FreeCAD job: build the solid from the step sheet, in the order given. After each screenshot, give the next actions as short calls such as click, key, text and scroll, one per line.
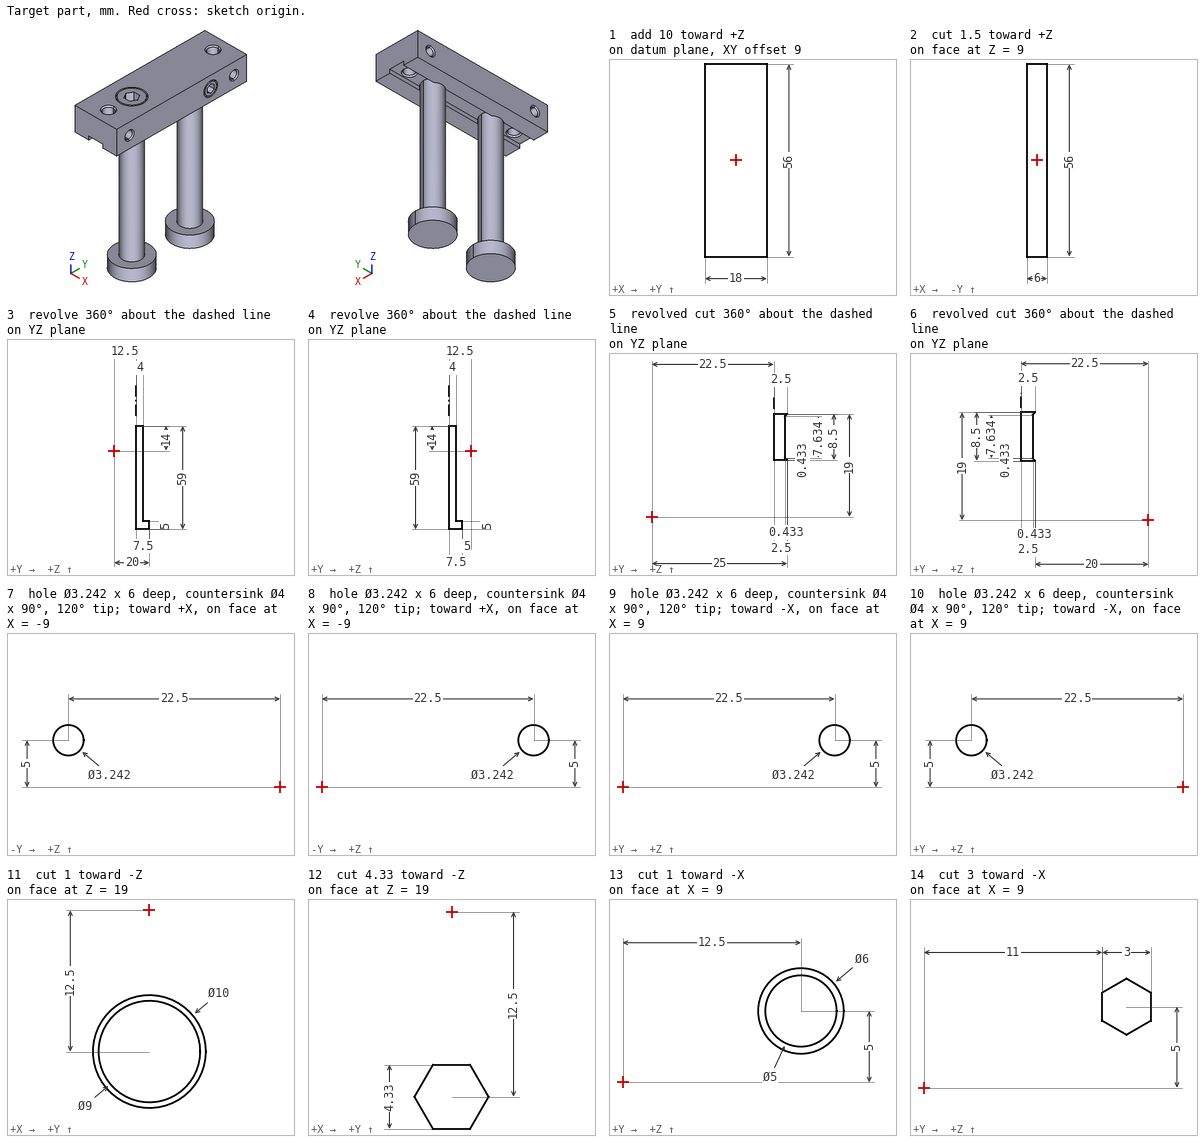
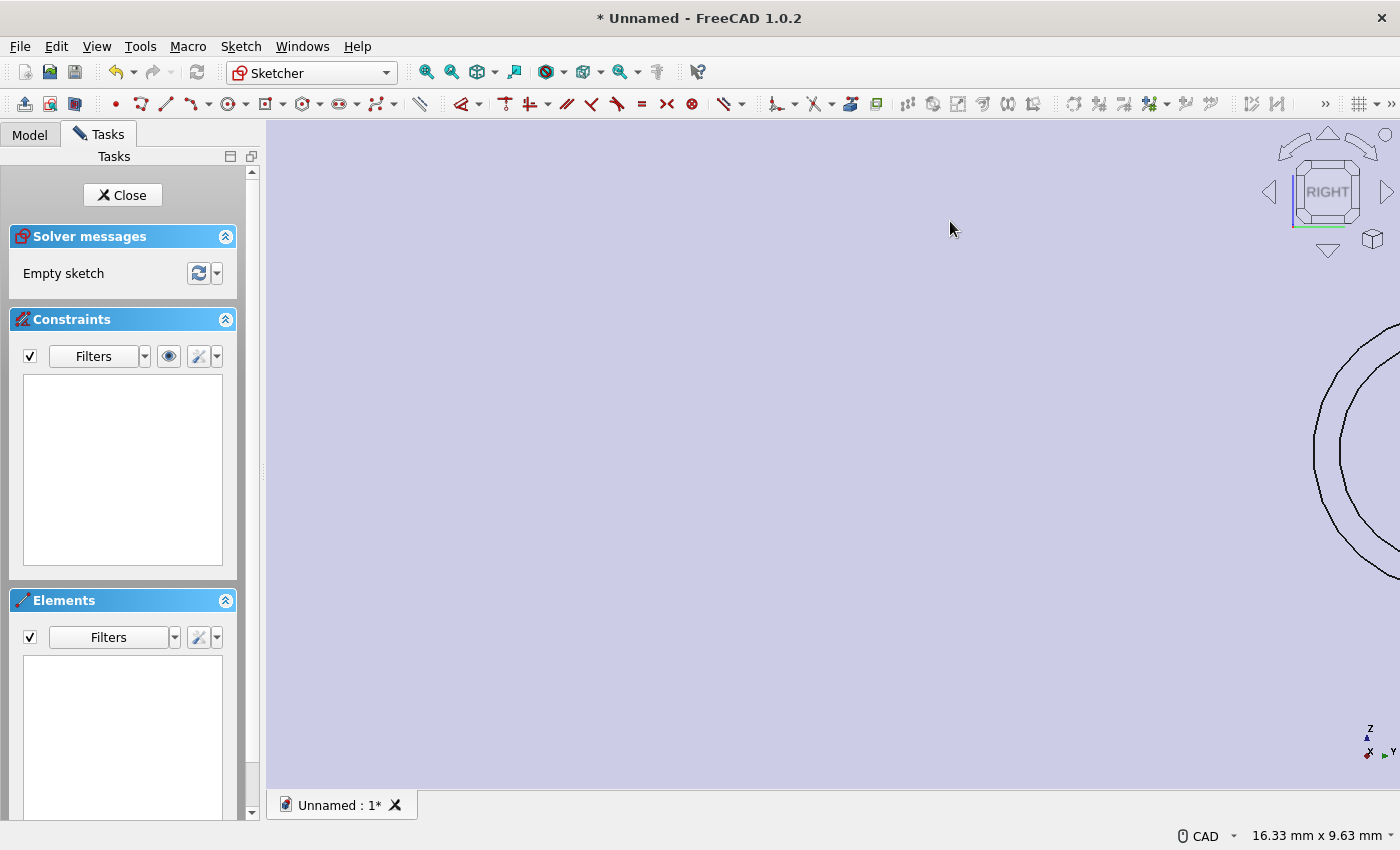
click(228, 104)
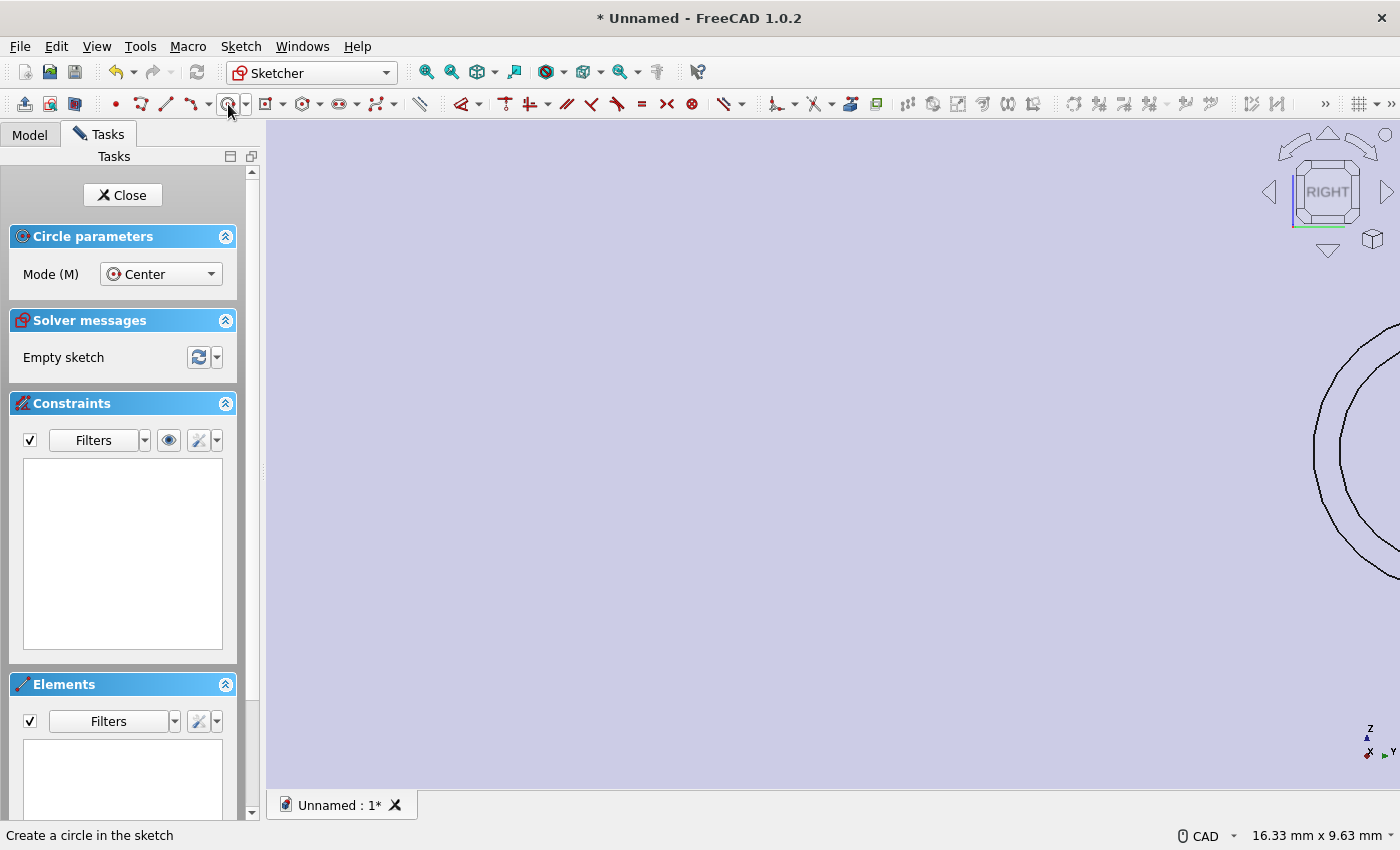
click(757, 452)
move(905, 304)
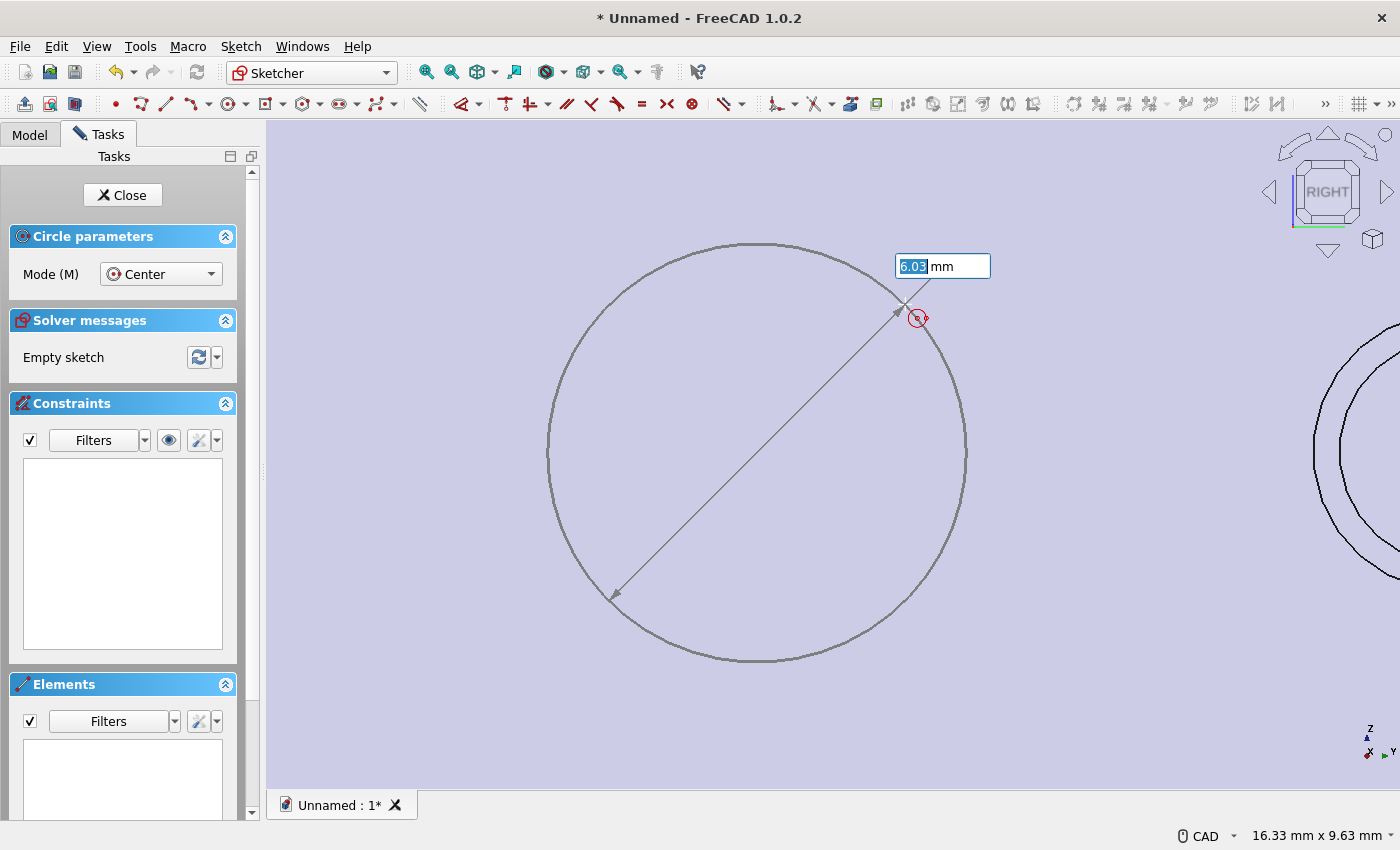
text(6)
key(Return)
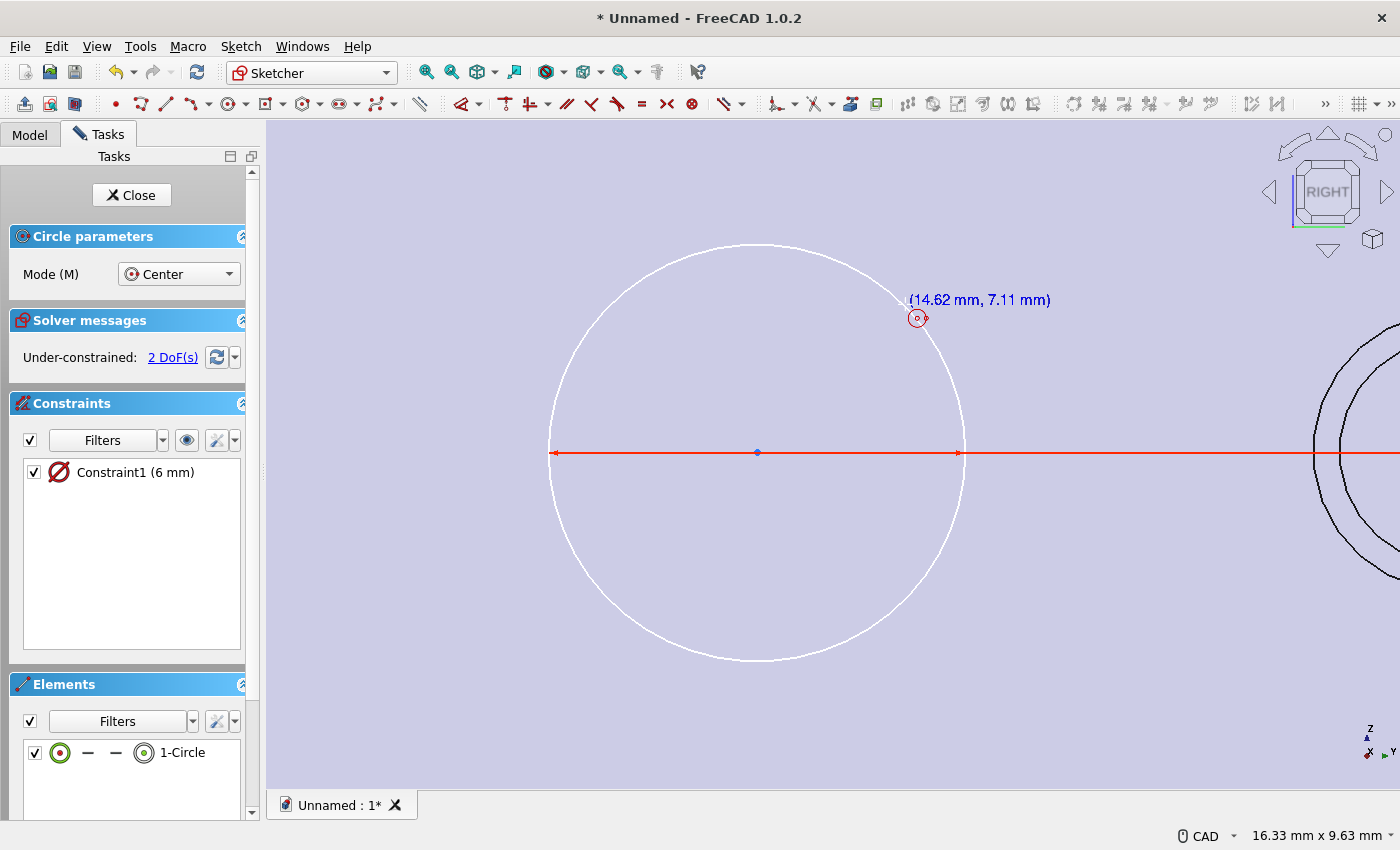
click(757, 453)
move(880, 329)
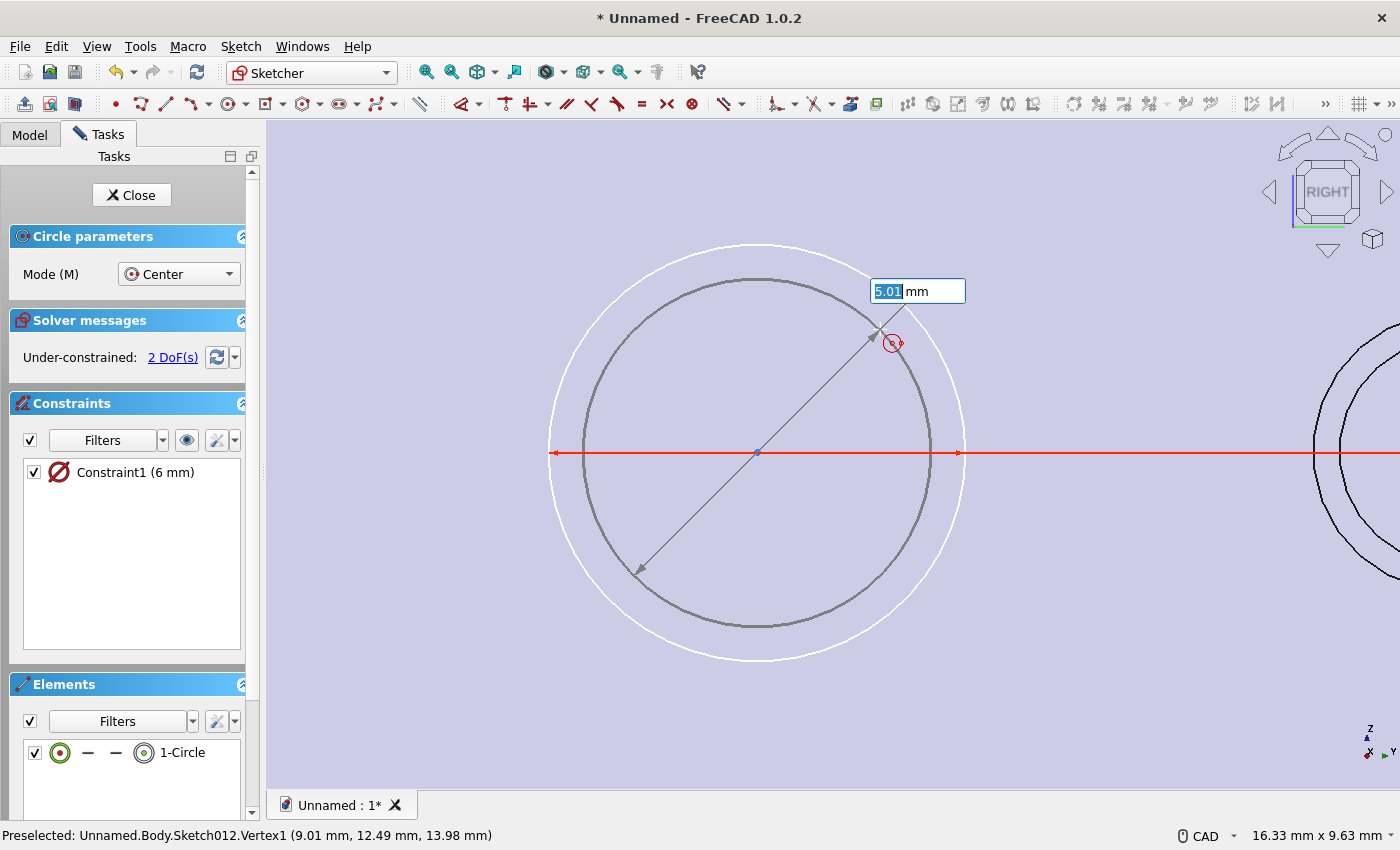
text(5)
key(Return)
key(Escape)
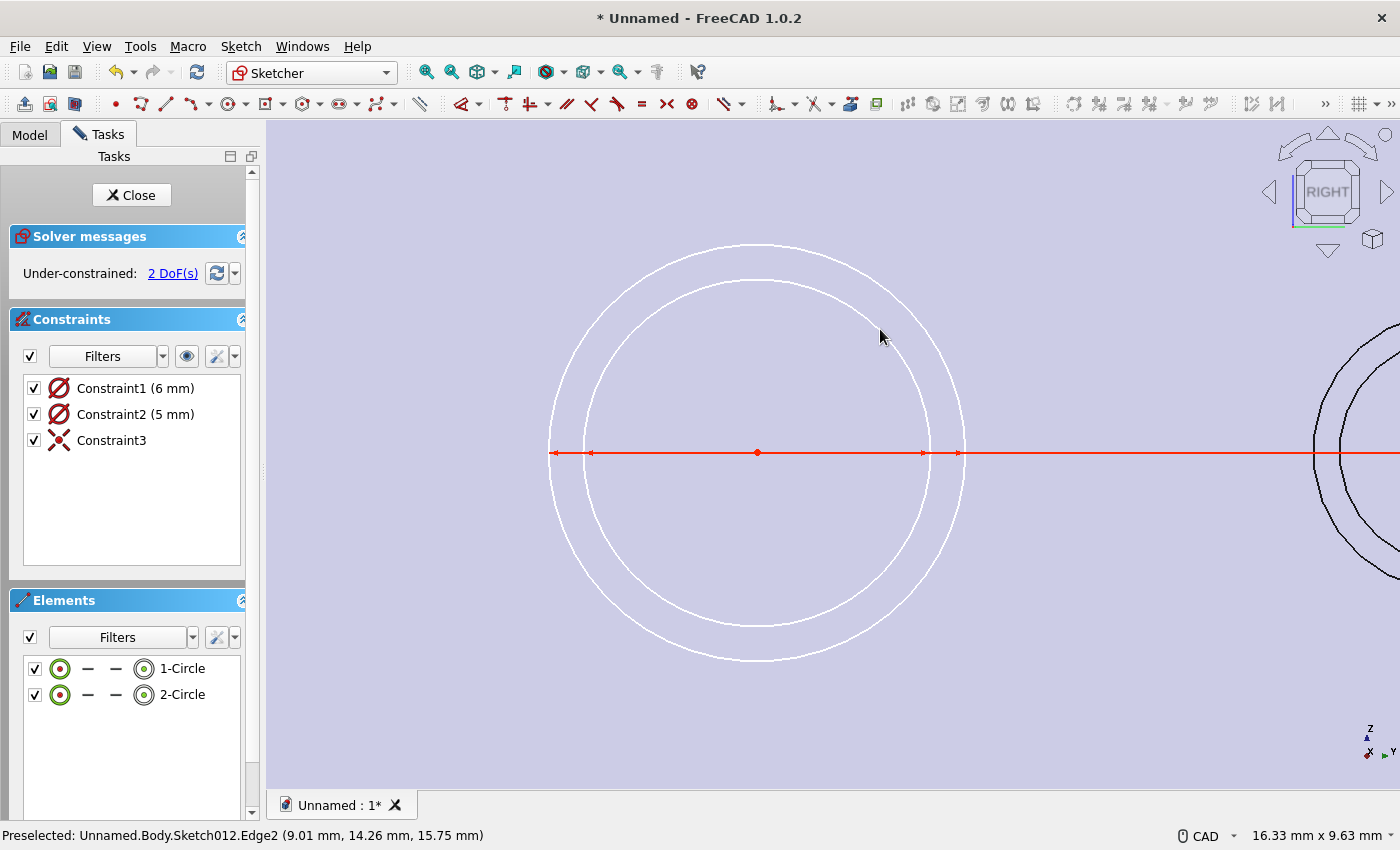
click(460, 104)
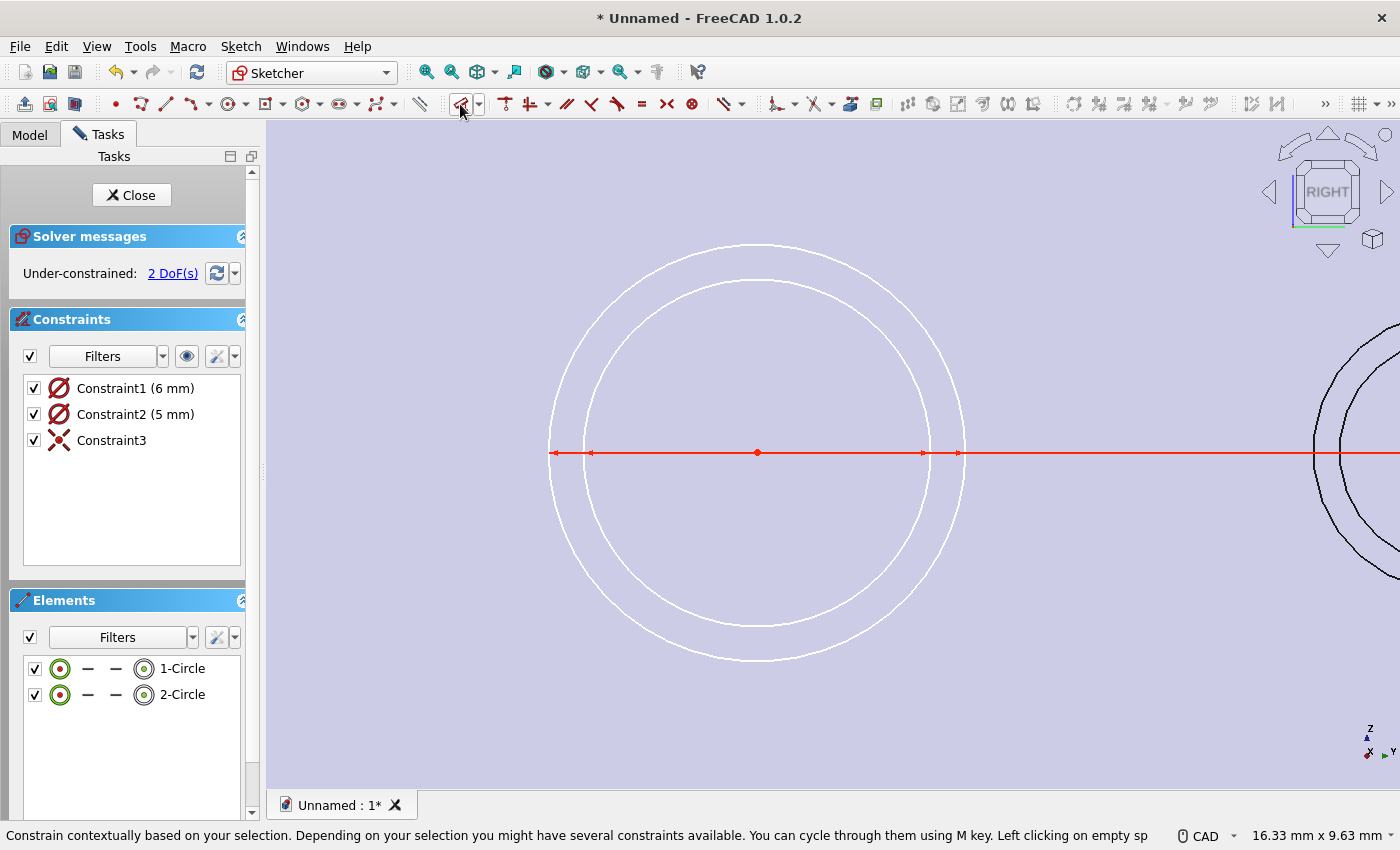
click(757, 453)
click(791, 607)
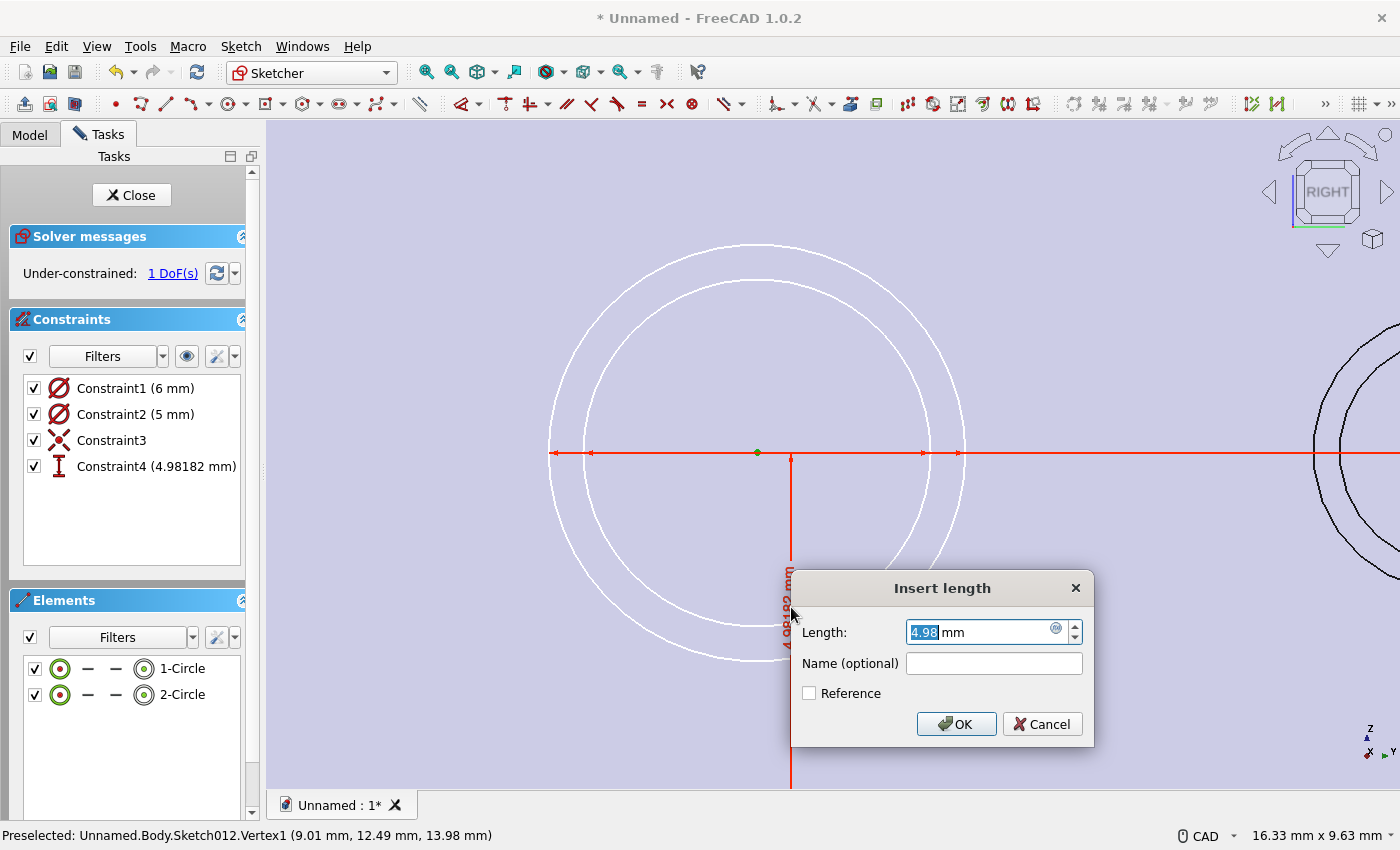
text(5)
key(Return)